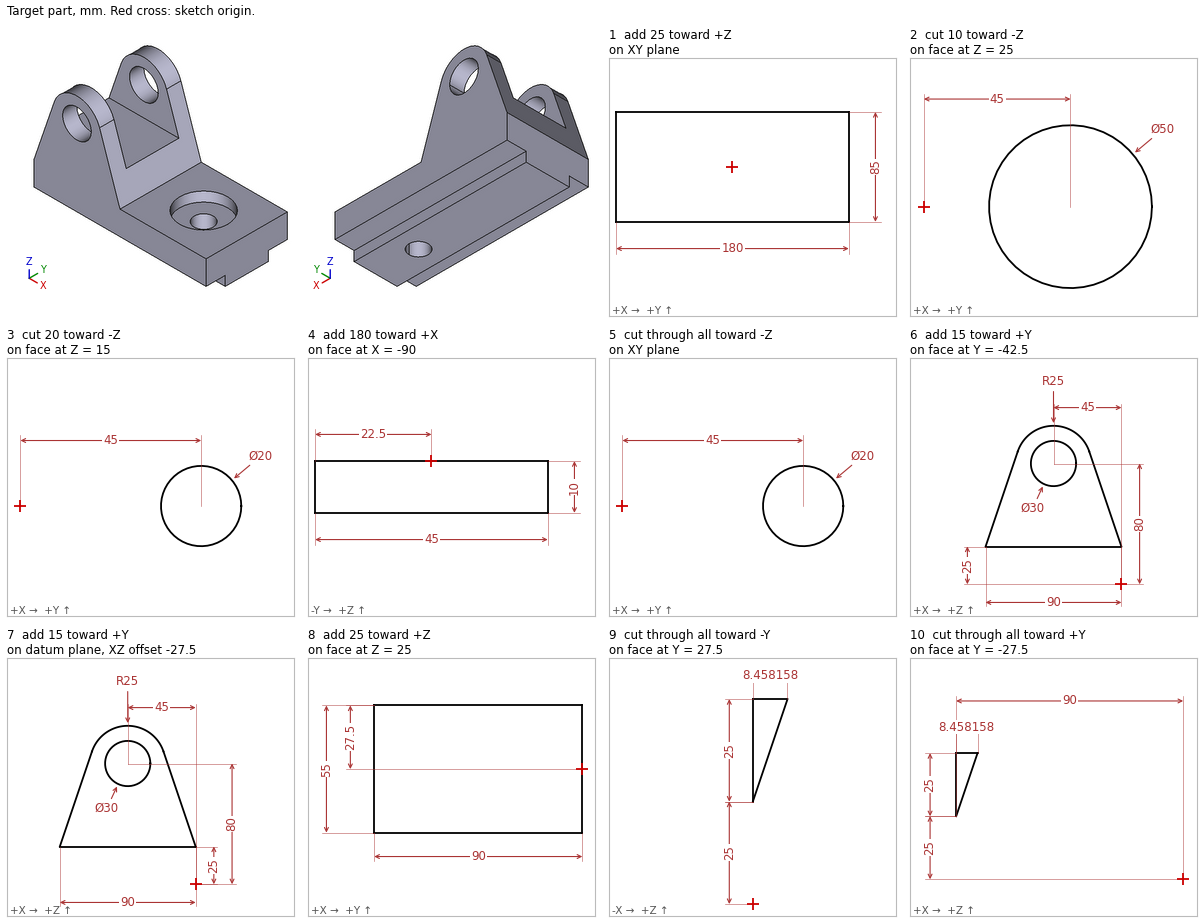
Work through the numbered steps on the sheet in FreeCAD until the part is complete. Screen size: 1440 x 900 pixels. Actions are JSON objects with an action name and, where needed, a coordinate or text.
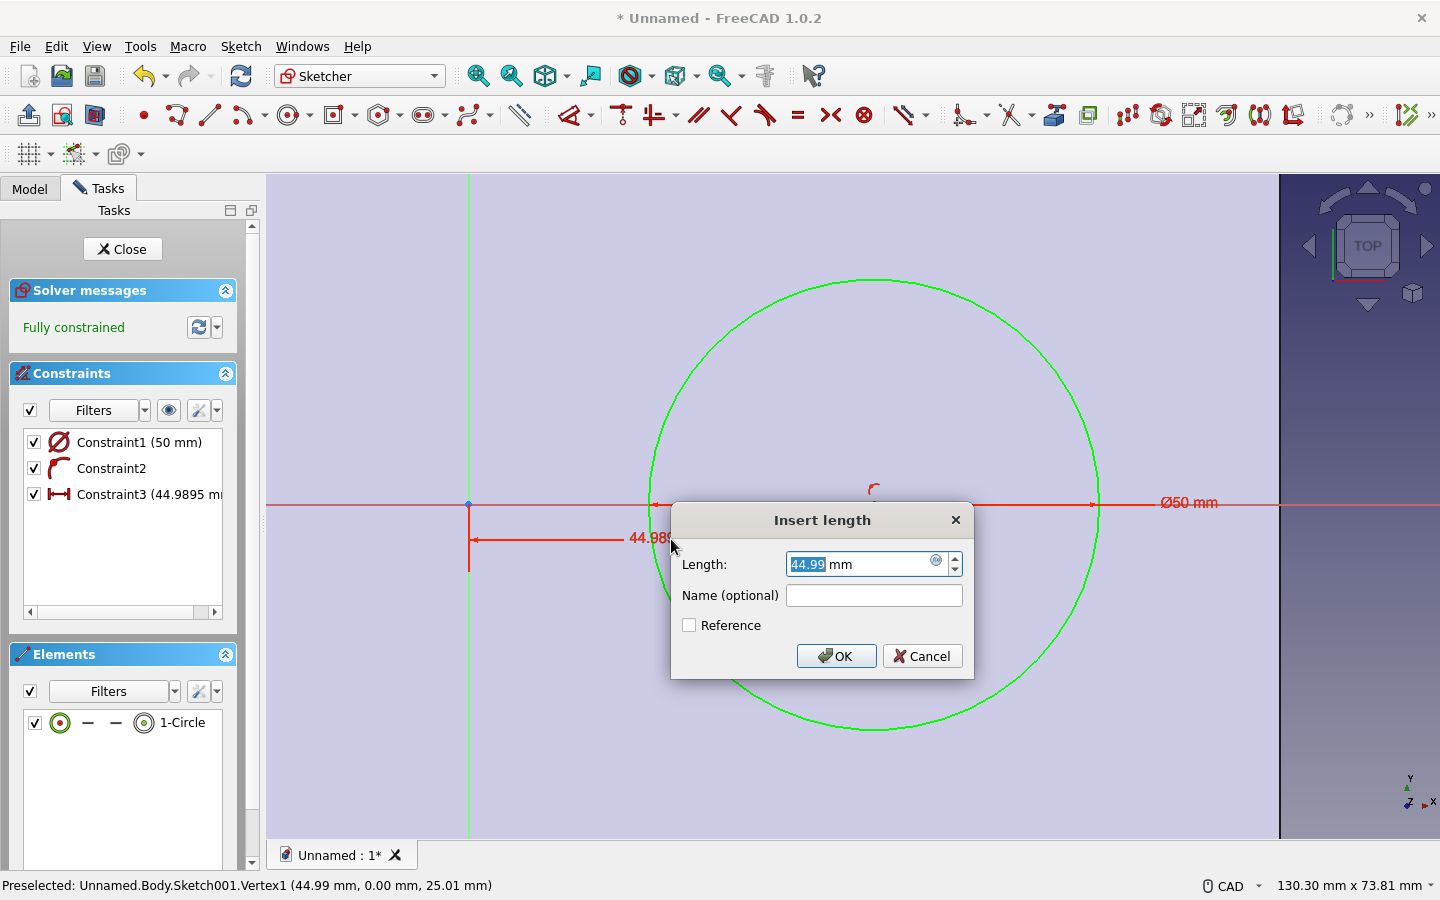
{"action": "type", "text": "45"}
{"action": "key", "text": "Return"}
{"action": "key", "text": "Escape"}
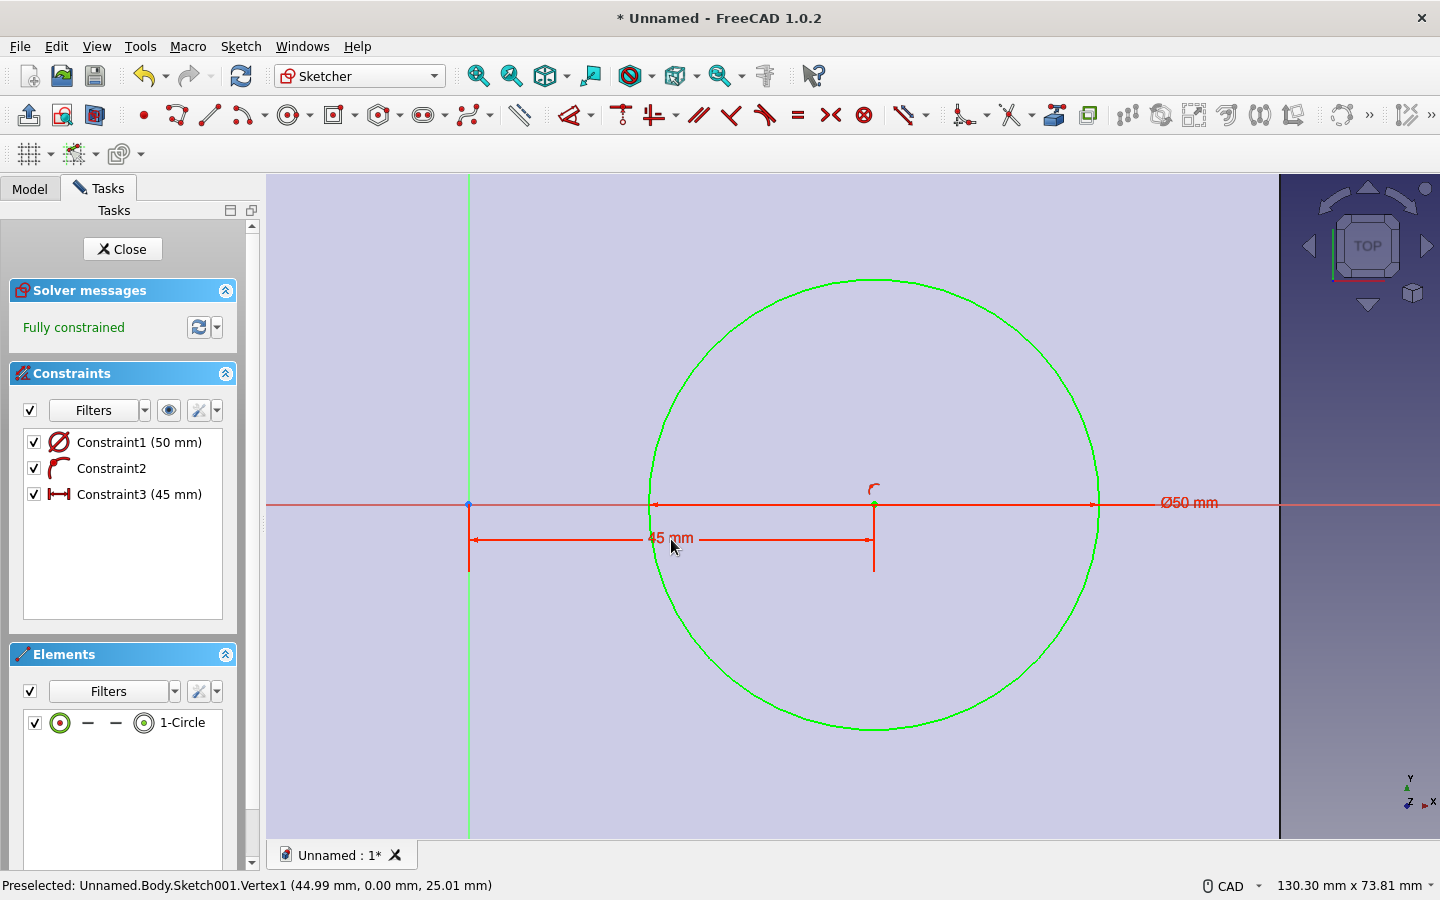
{"action": "left_click", "coordinate": [123, 249]}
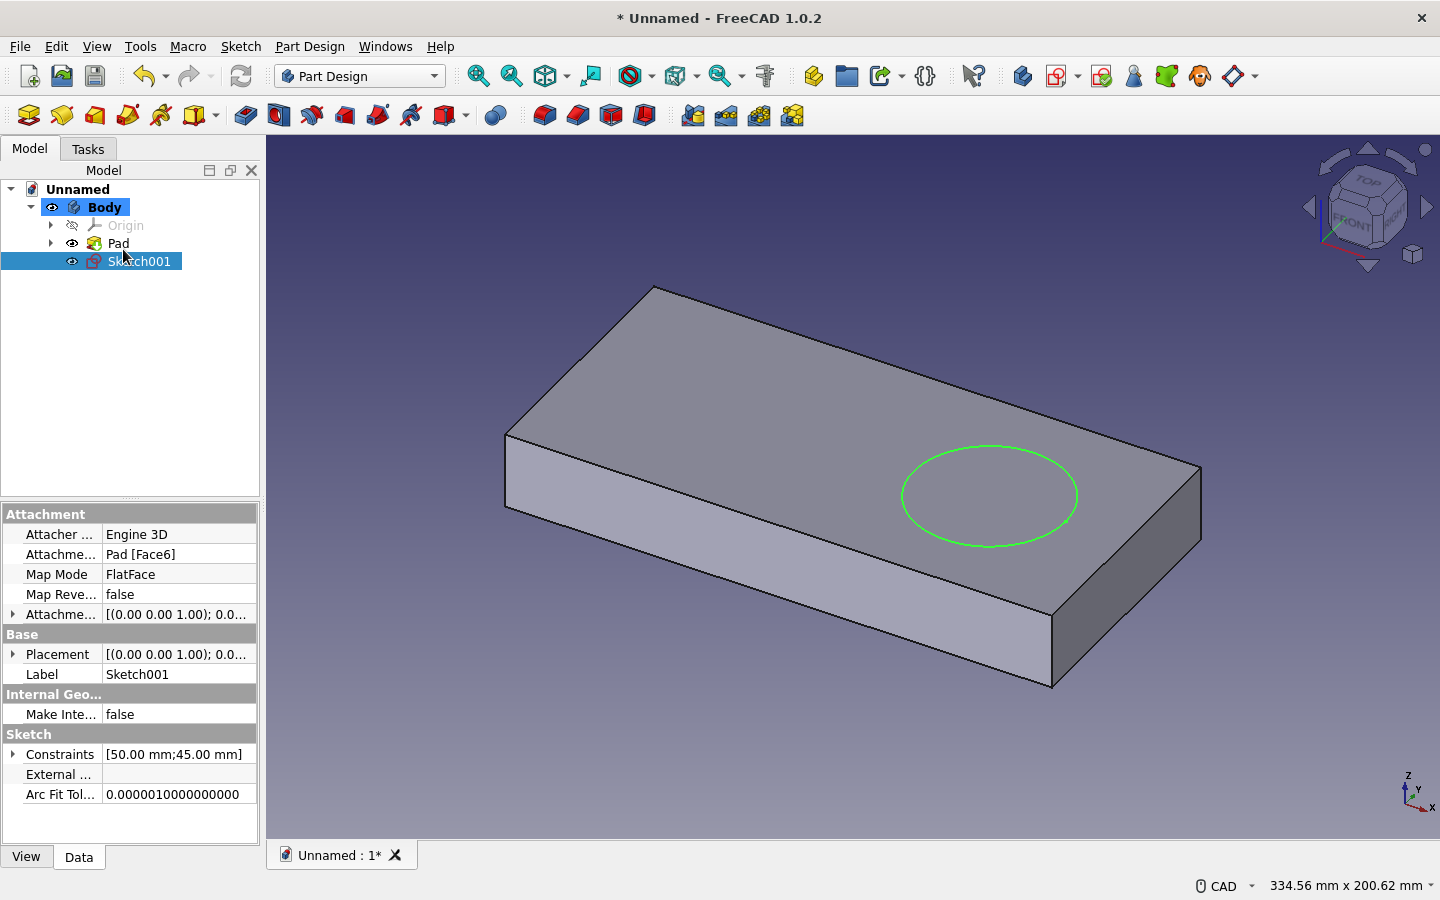
{"action": "left_click", "coordinate": [246, 116]}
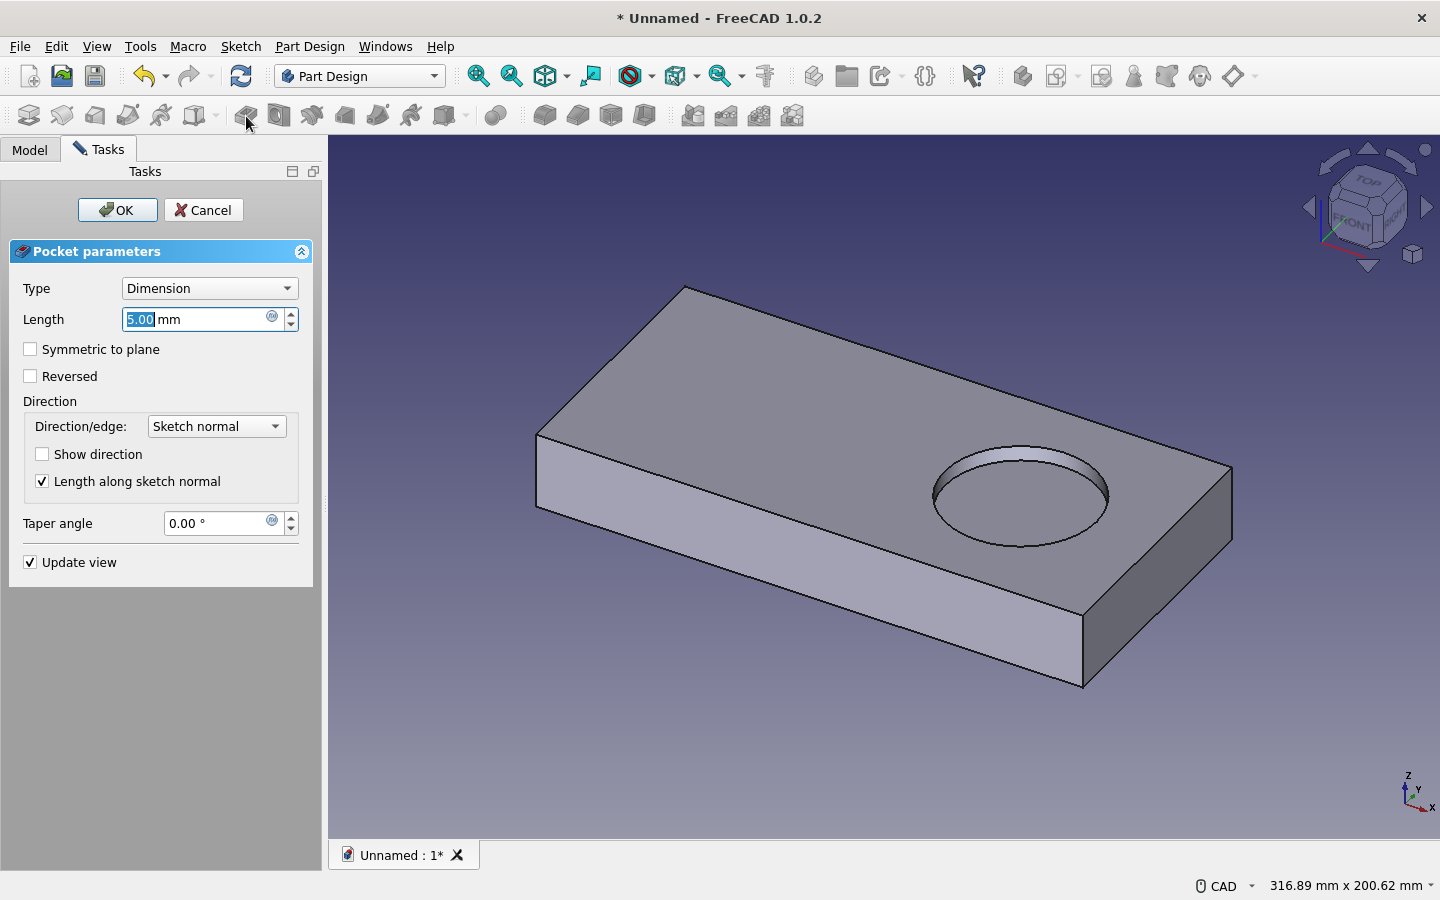
{"action": "type", "text": "10"}
{"action": "key", "text": "Tab"}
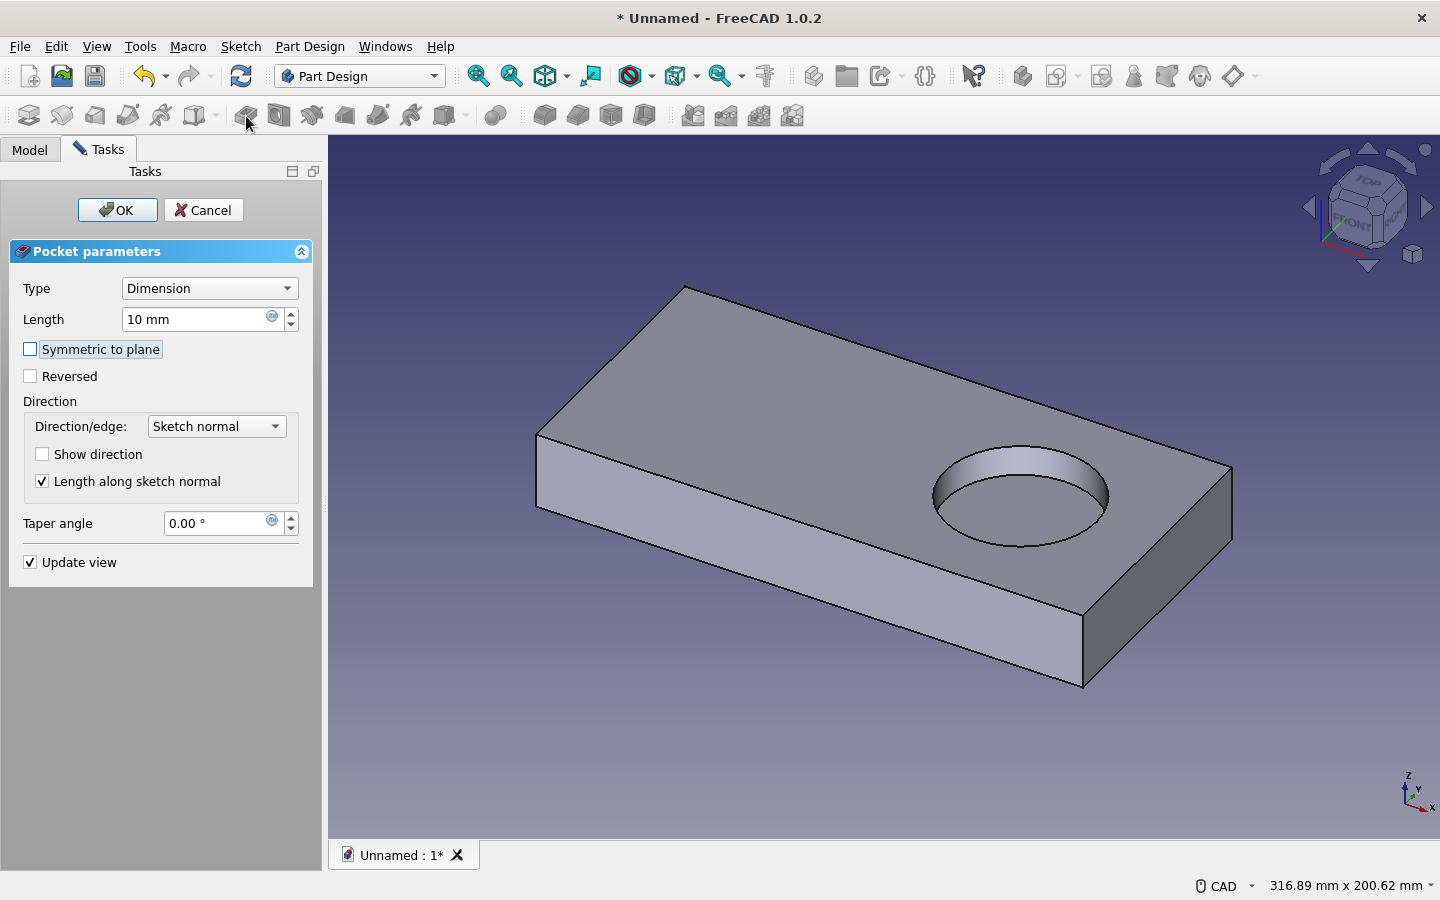
{"action": "left_click", "coordinate": [118, 210]}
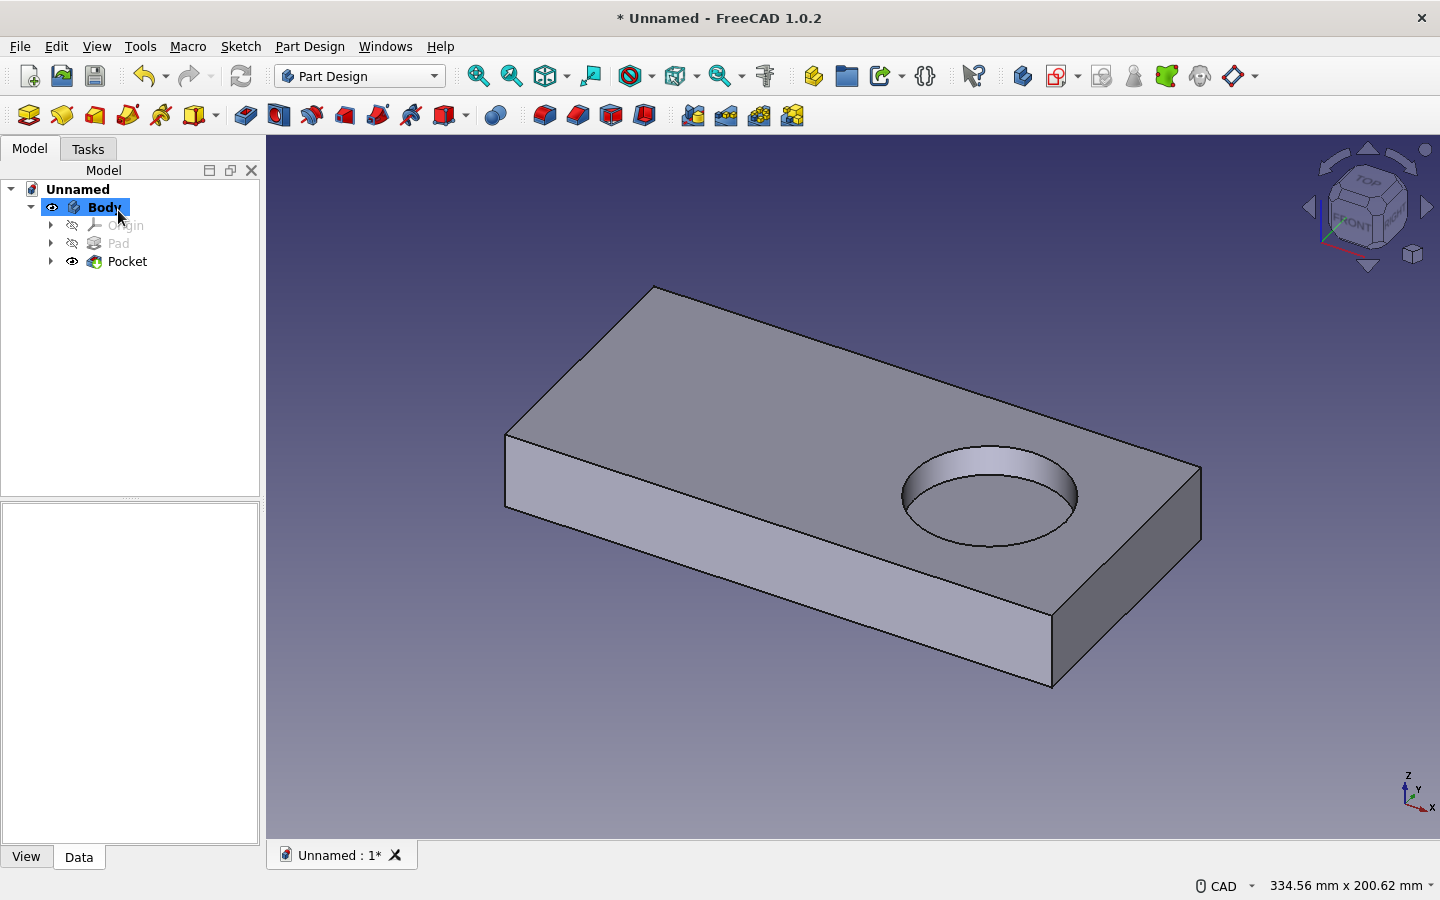
{"action": "left_click", "coordinate": [990, 524]}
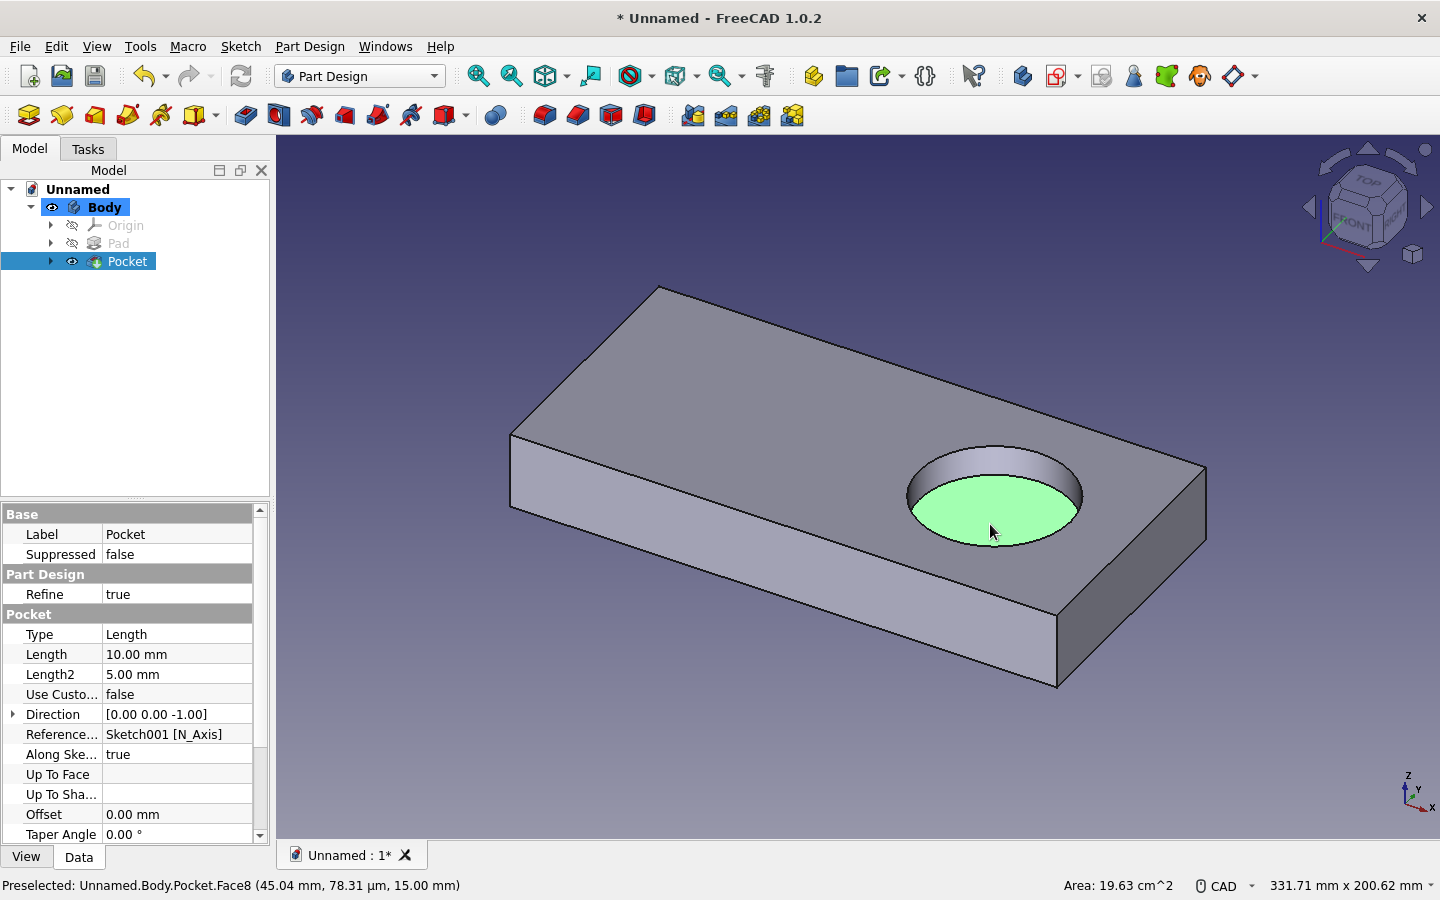
{"action": "left_click", "coordinate": [1056, 76]}